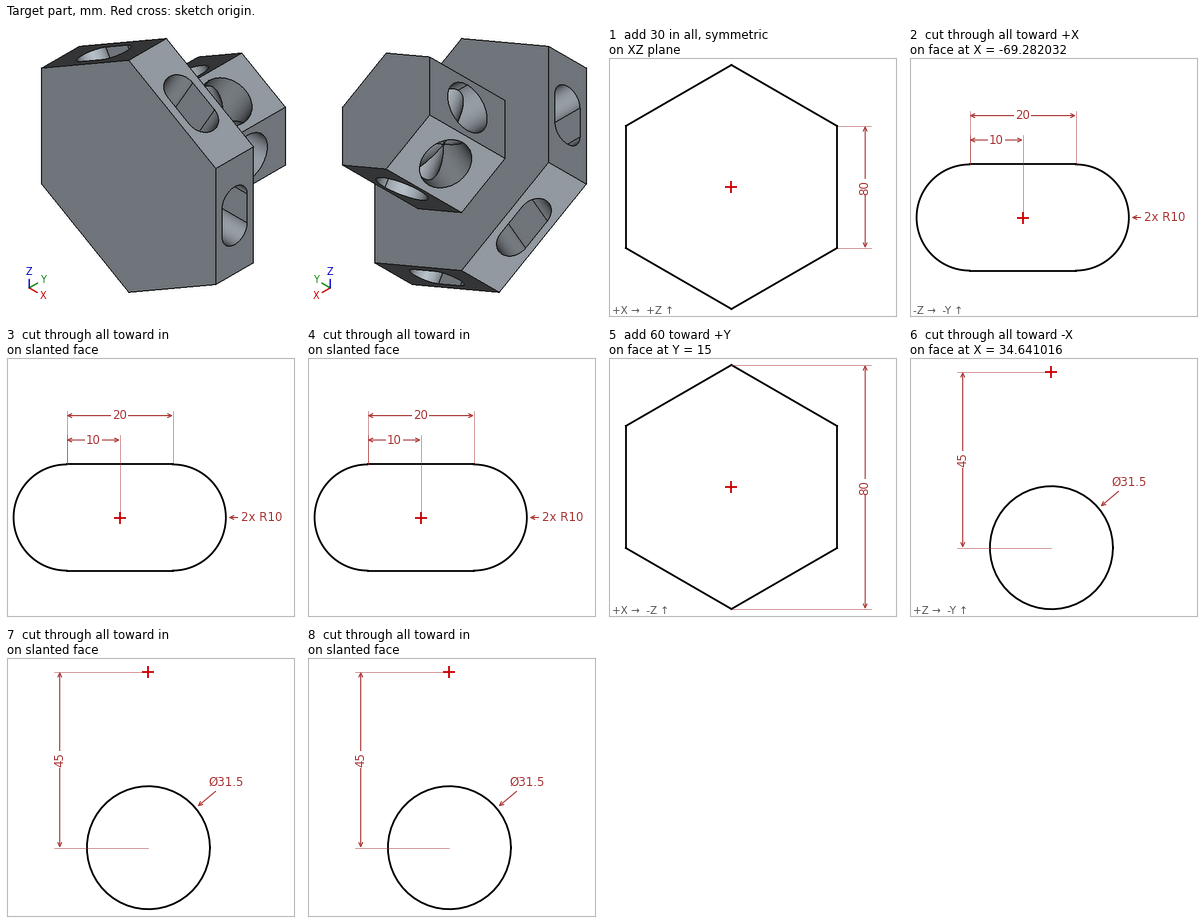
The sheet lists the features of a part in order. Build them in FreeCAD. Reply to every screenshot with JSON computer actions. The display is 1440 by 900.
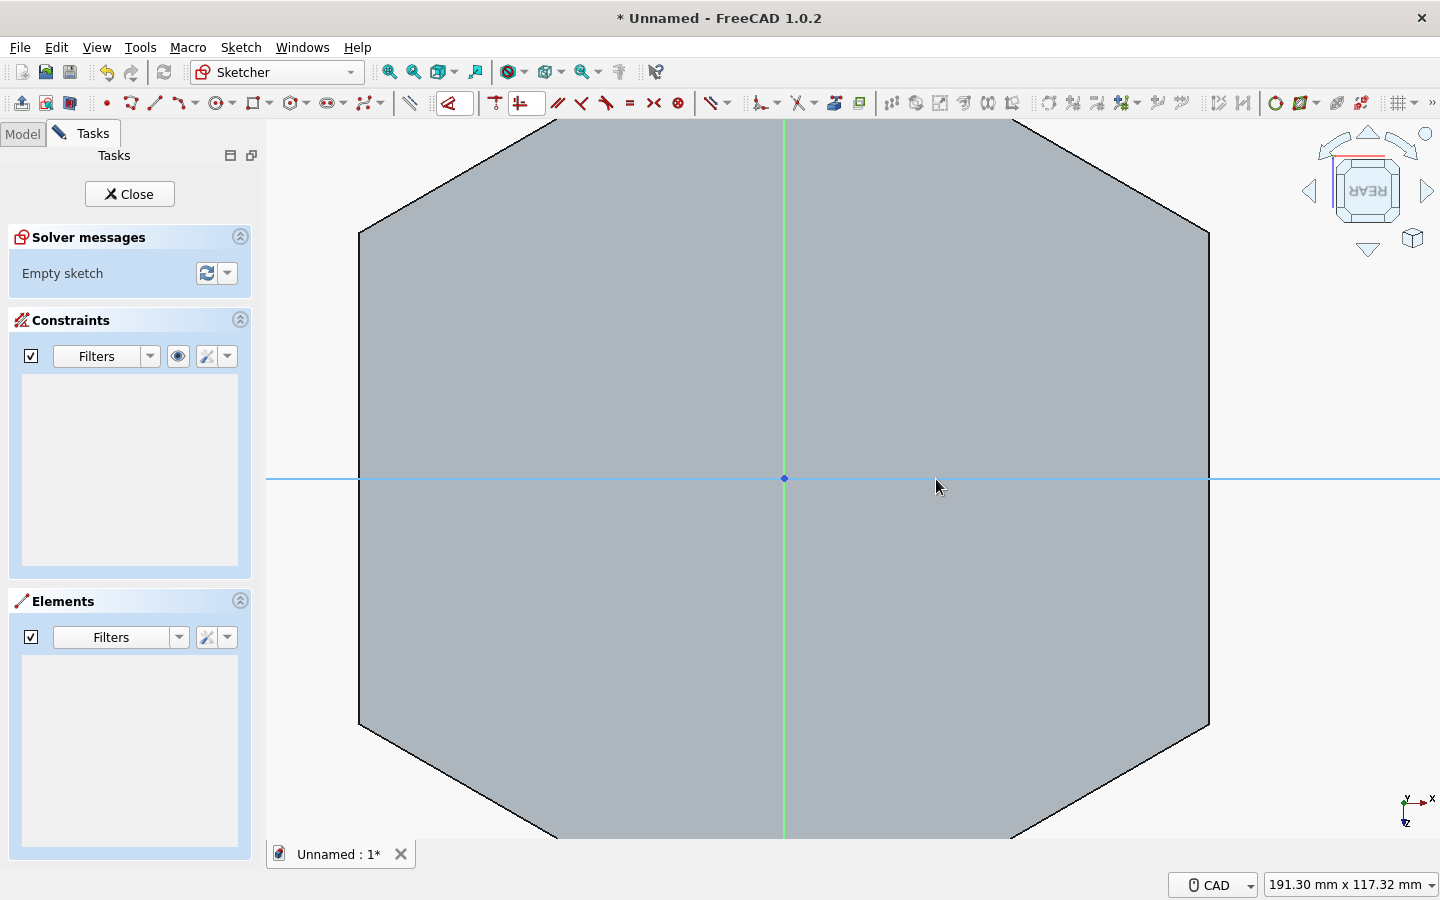
{"action": "left_click", "coordinate": [290, 104]}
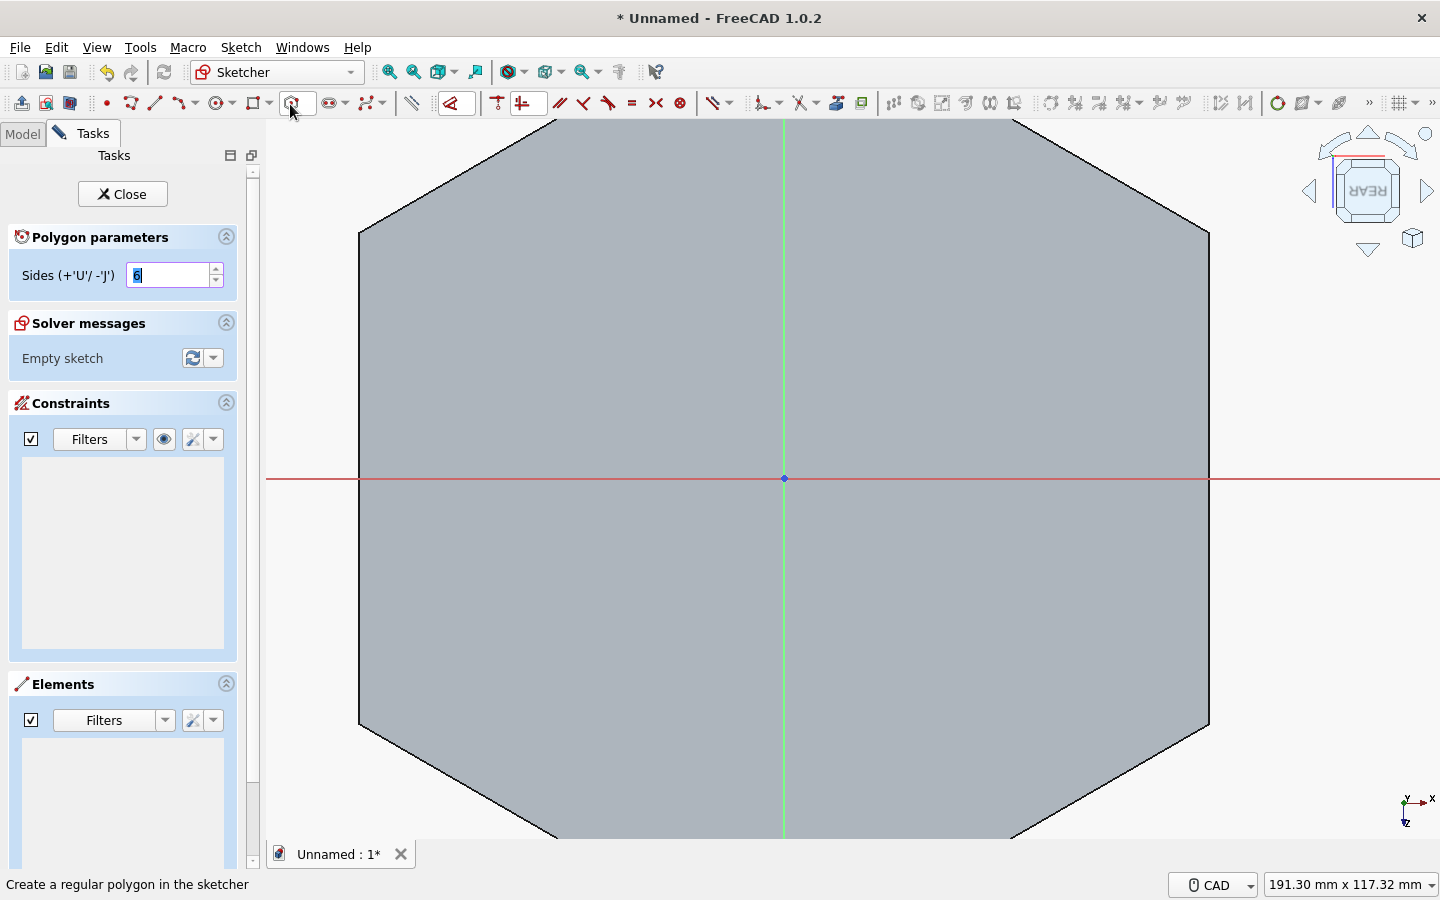
{"action": "left_click", "coordinate": [784, 479]}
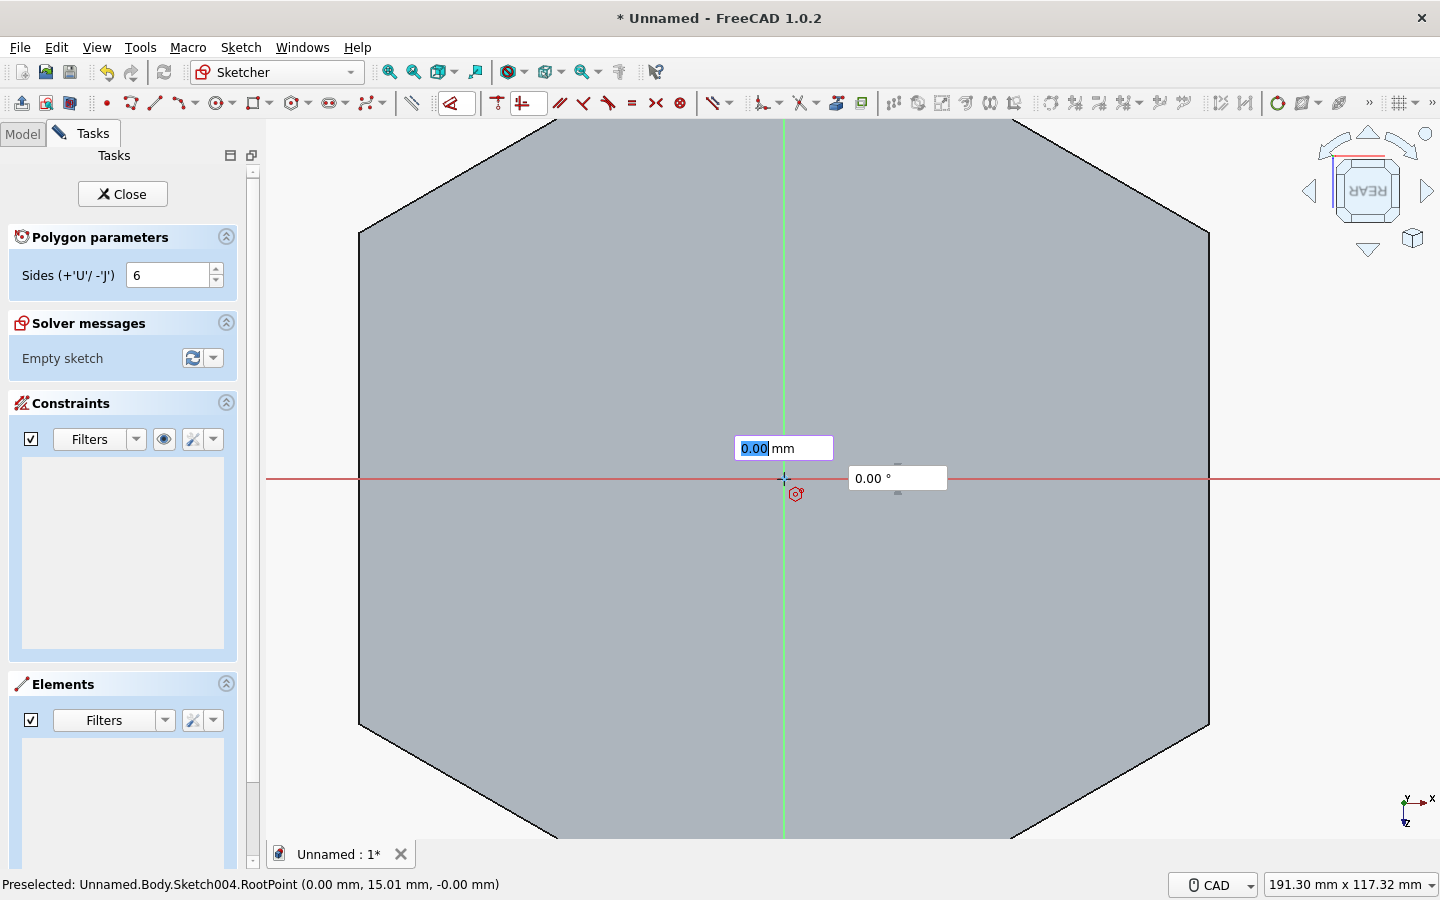
{"action": "left_click", "coordinate": [784, 233]}
{"action": "right_click", "coordinate": [784, 233]}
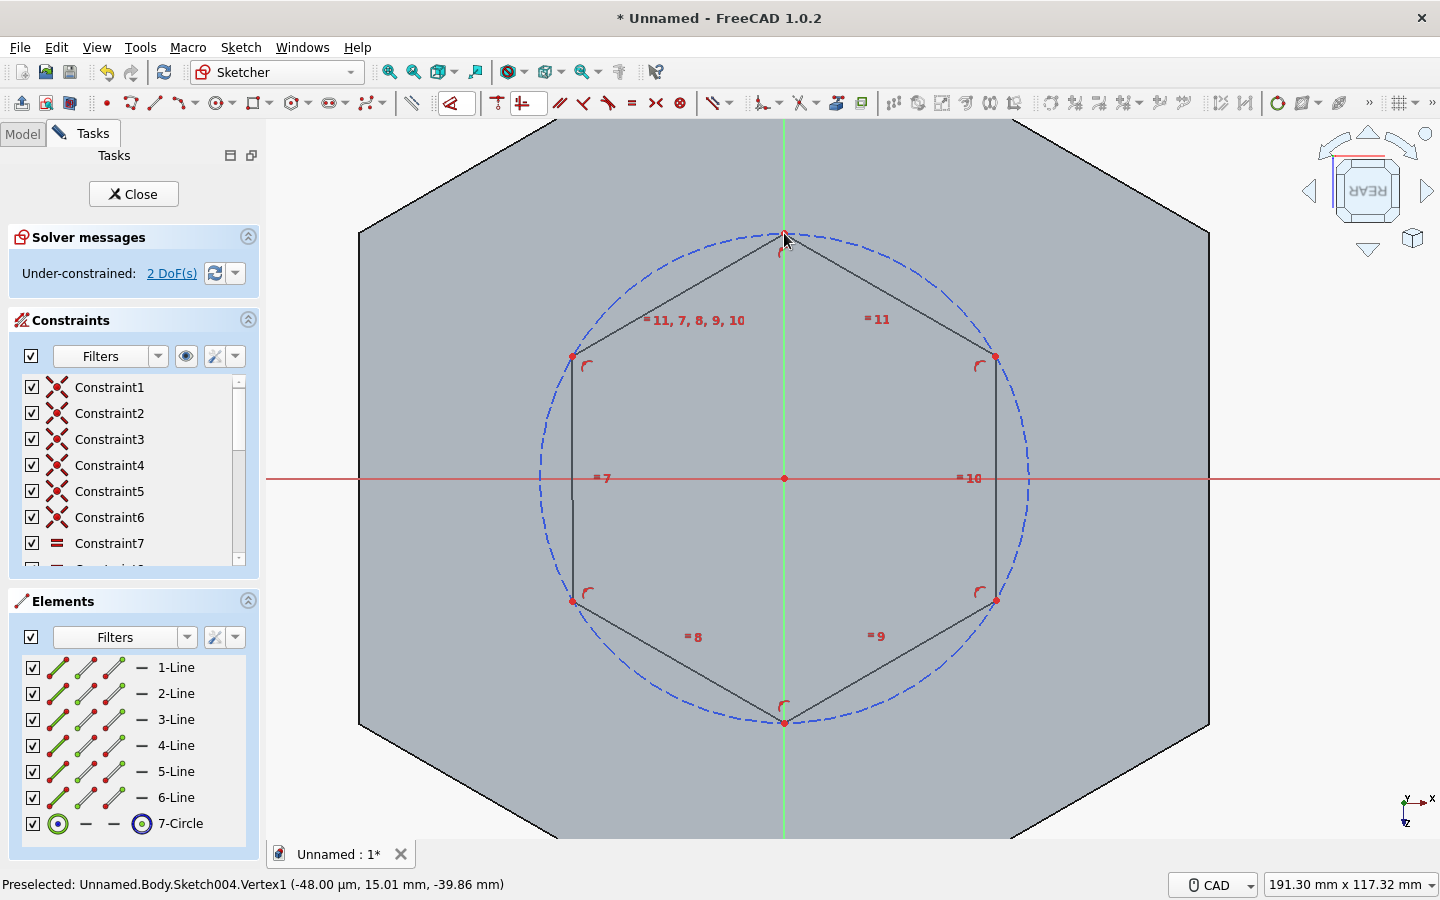
{"action": "left_click", "coordinate": [572, 430]}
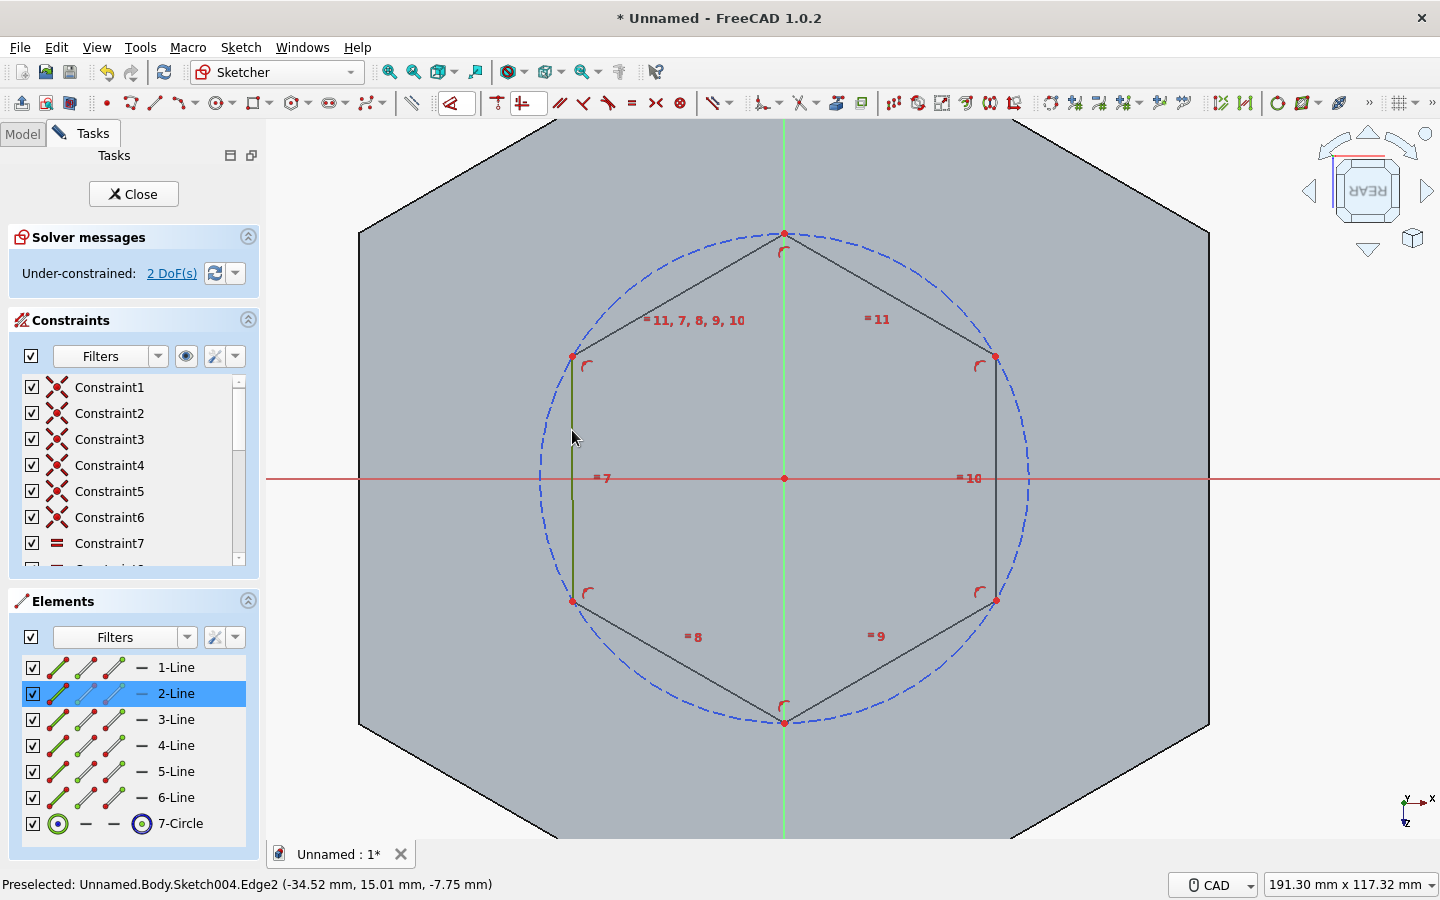
{"action": "left_click", "coordinate": [542, 104]}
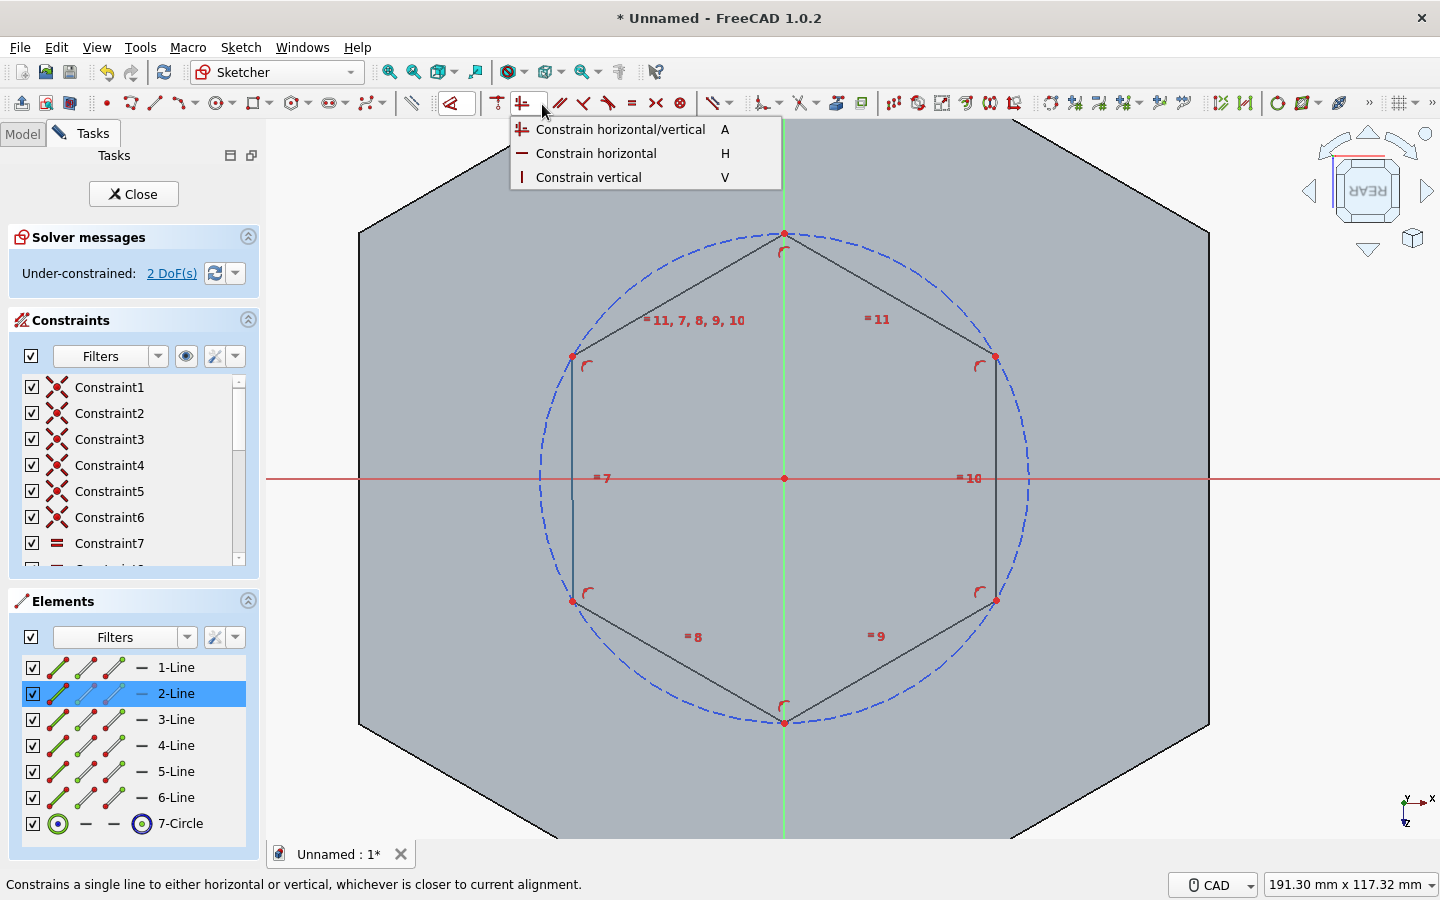
{"action": "left_click", "coordinate": [646, 177]}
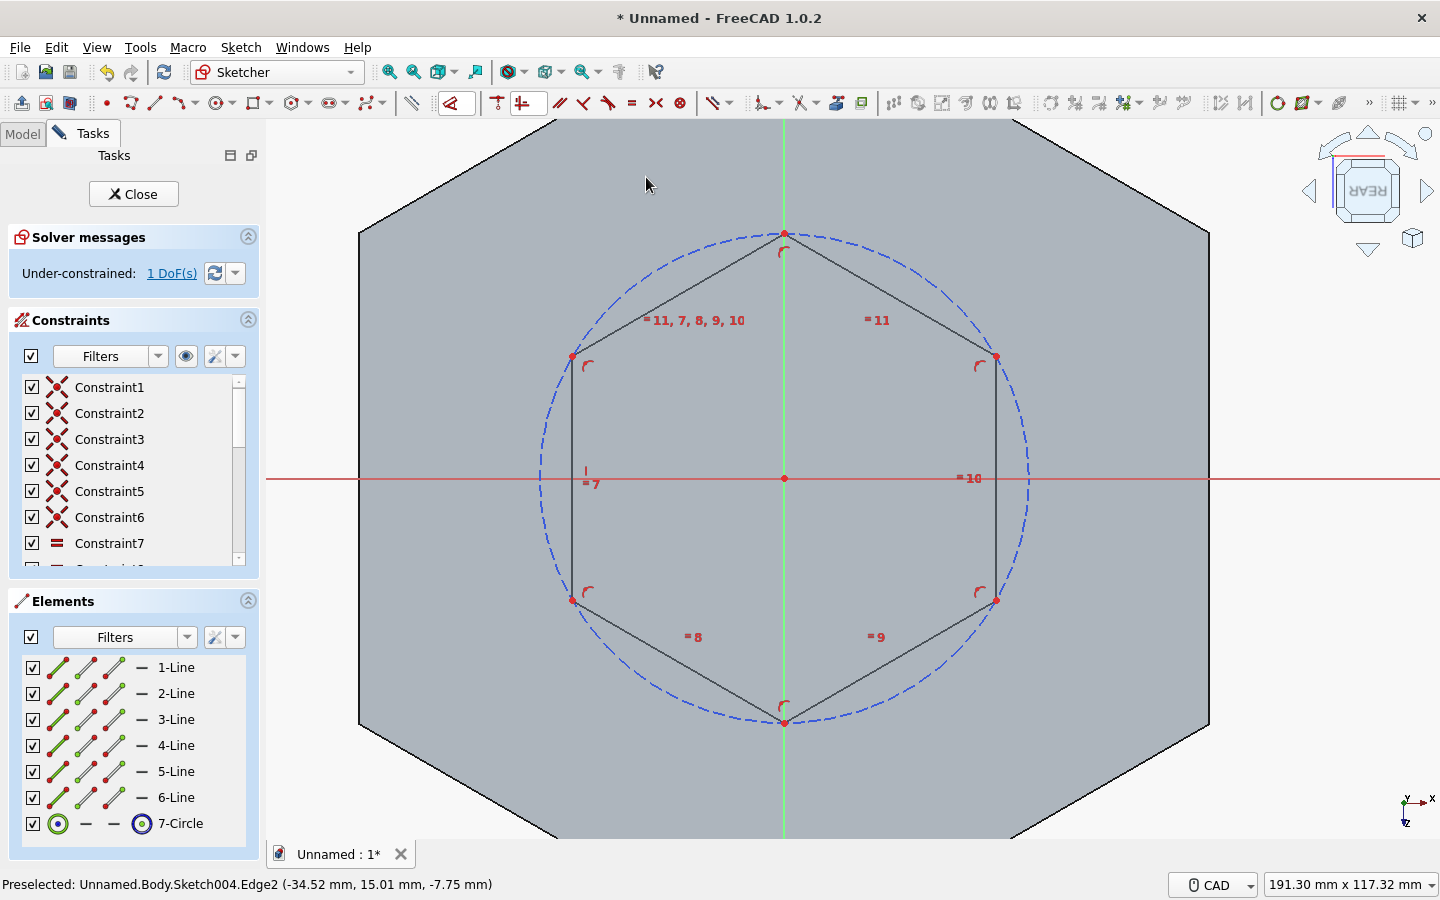
{"action": "left_click", "coordinate": [784, 723]}